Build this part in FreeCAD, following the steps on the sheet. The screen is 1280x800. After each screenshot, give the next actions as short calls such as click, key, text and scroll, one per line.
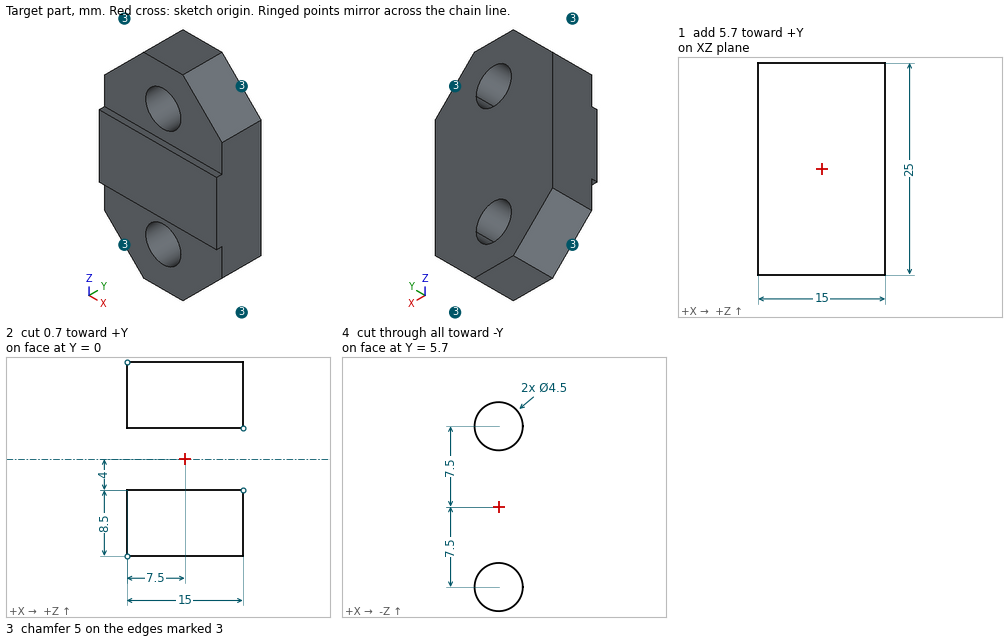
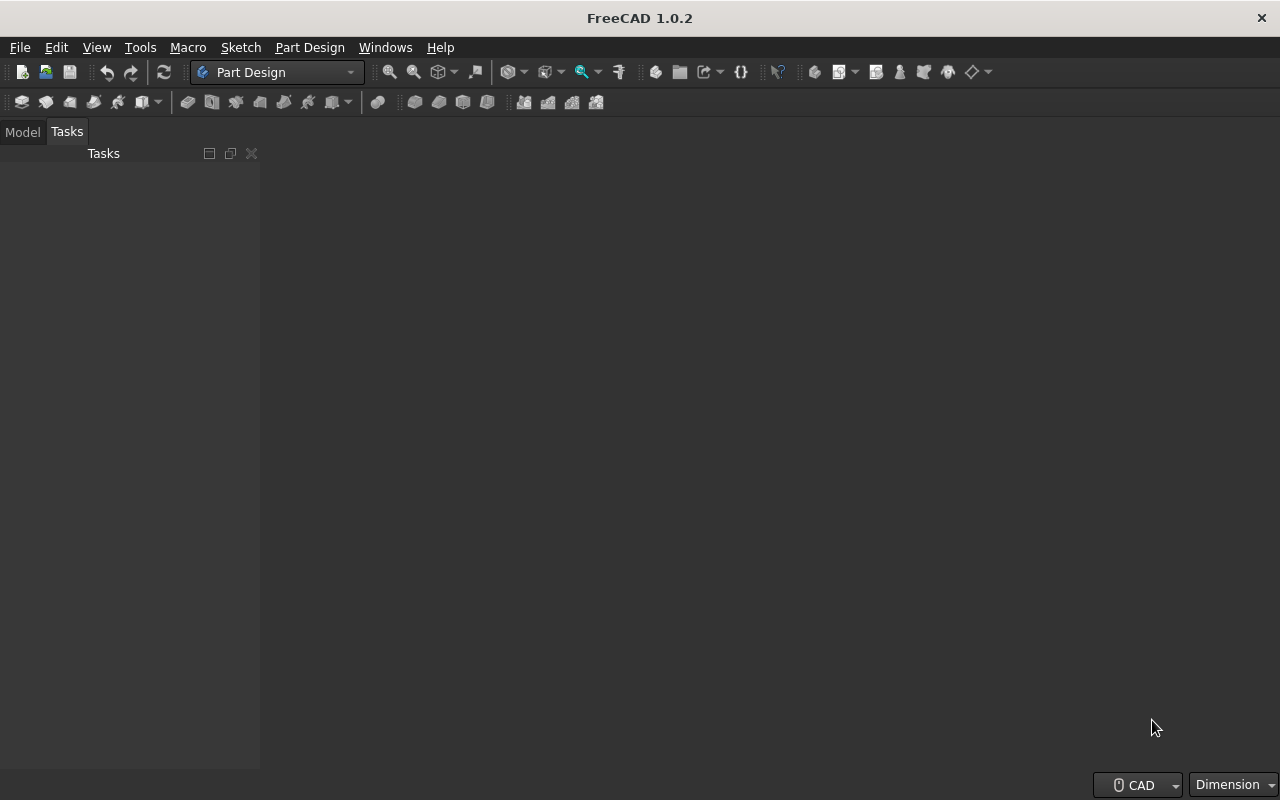
key(ctrl+n)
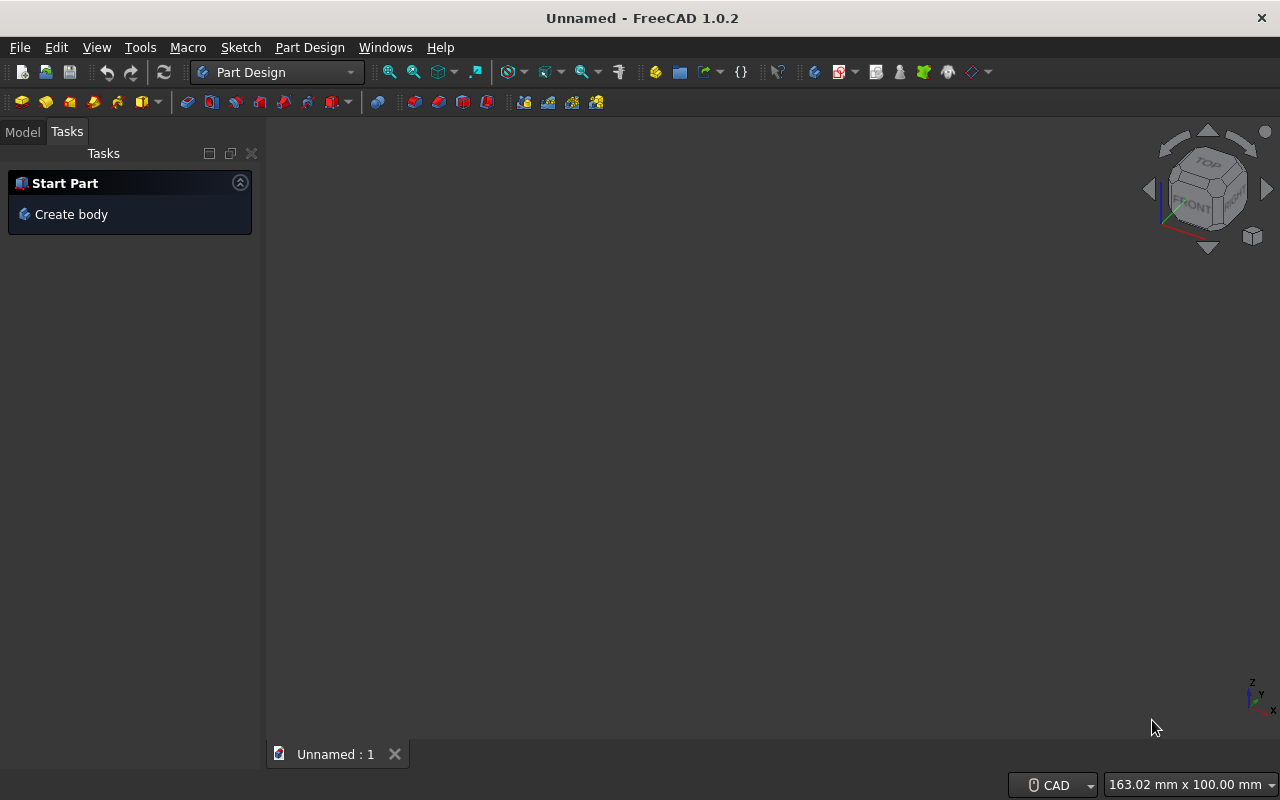
click(840, 72)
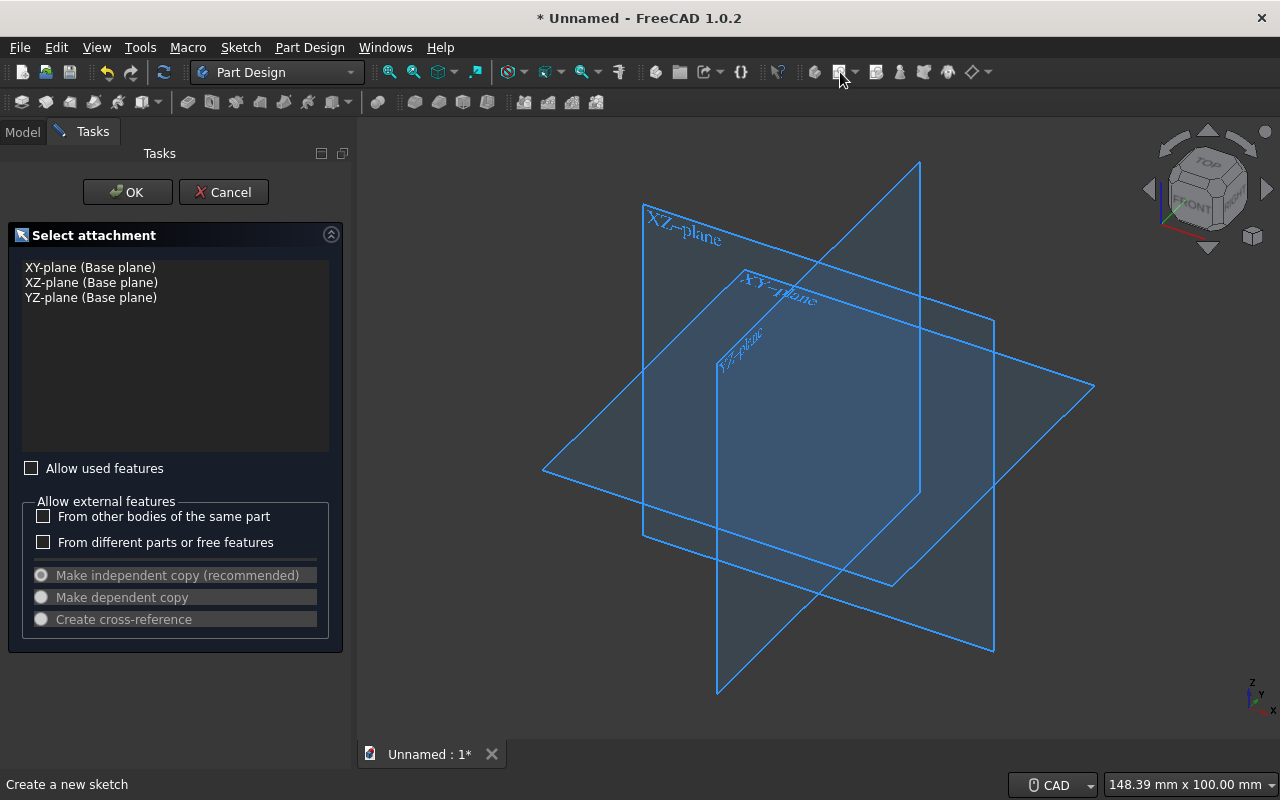
click(82, 282)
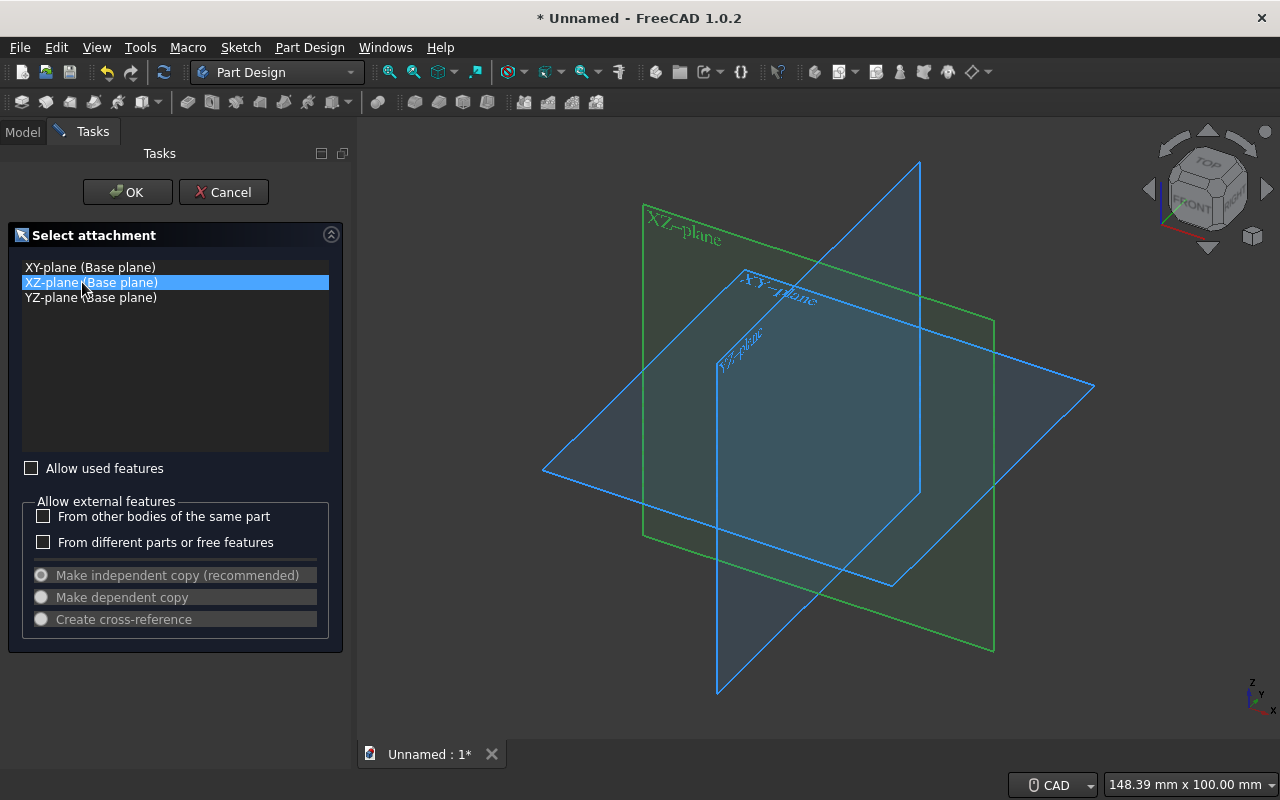
click(128, 192)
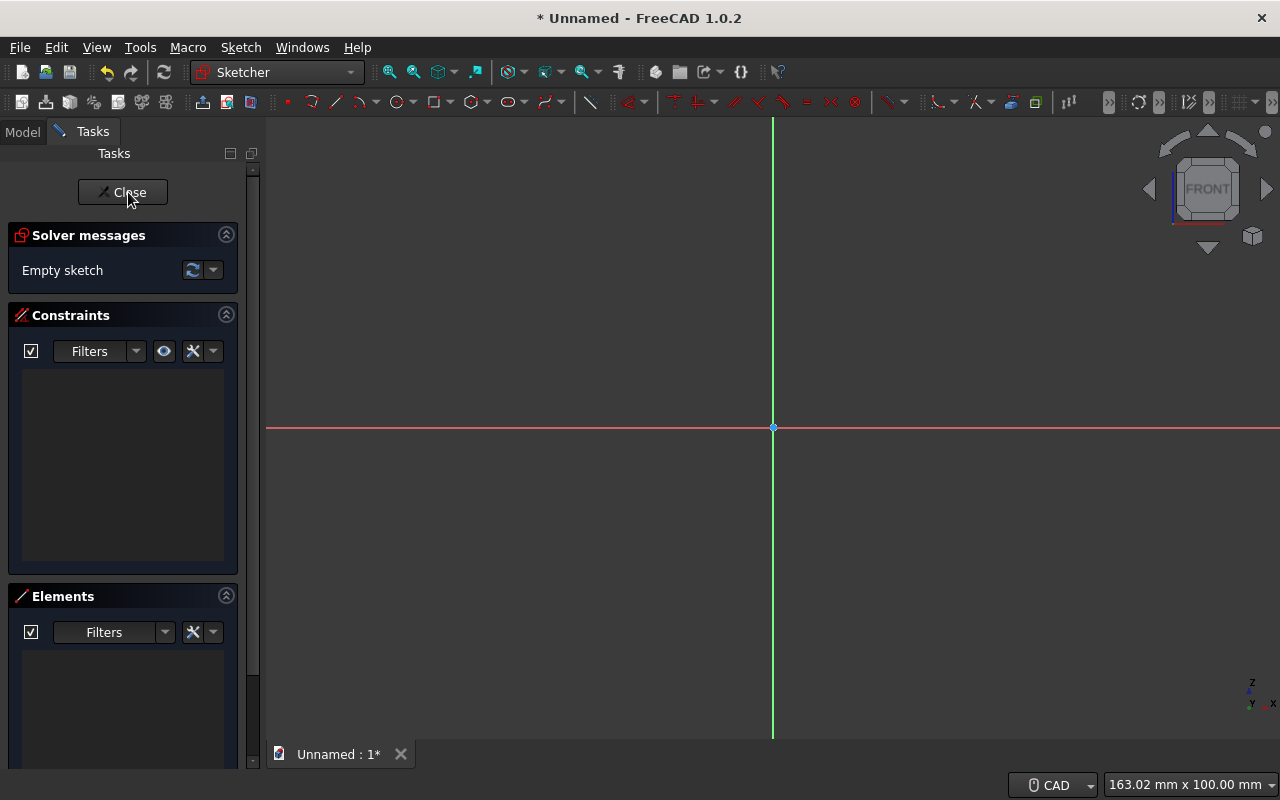
scroll(813, 428, up, 5)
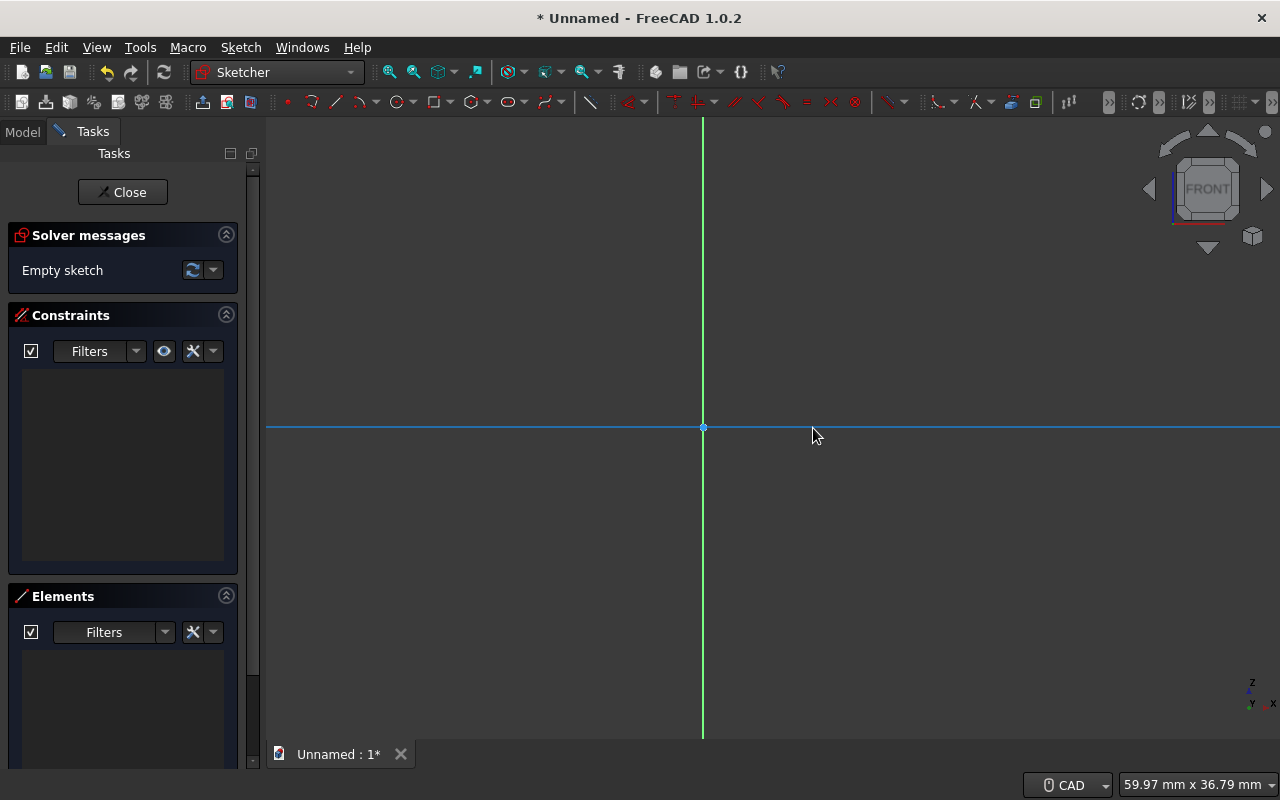
click(452, 102)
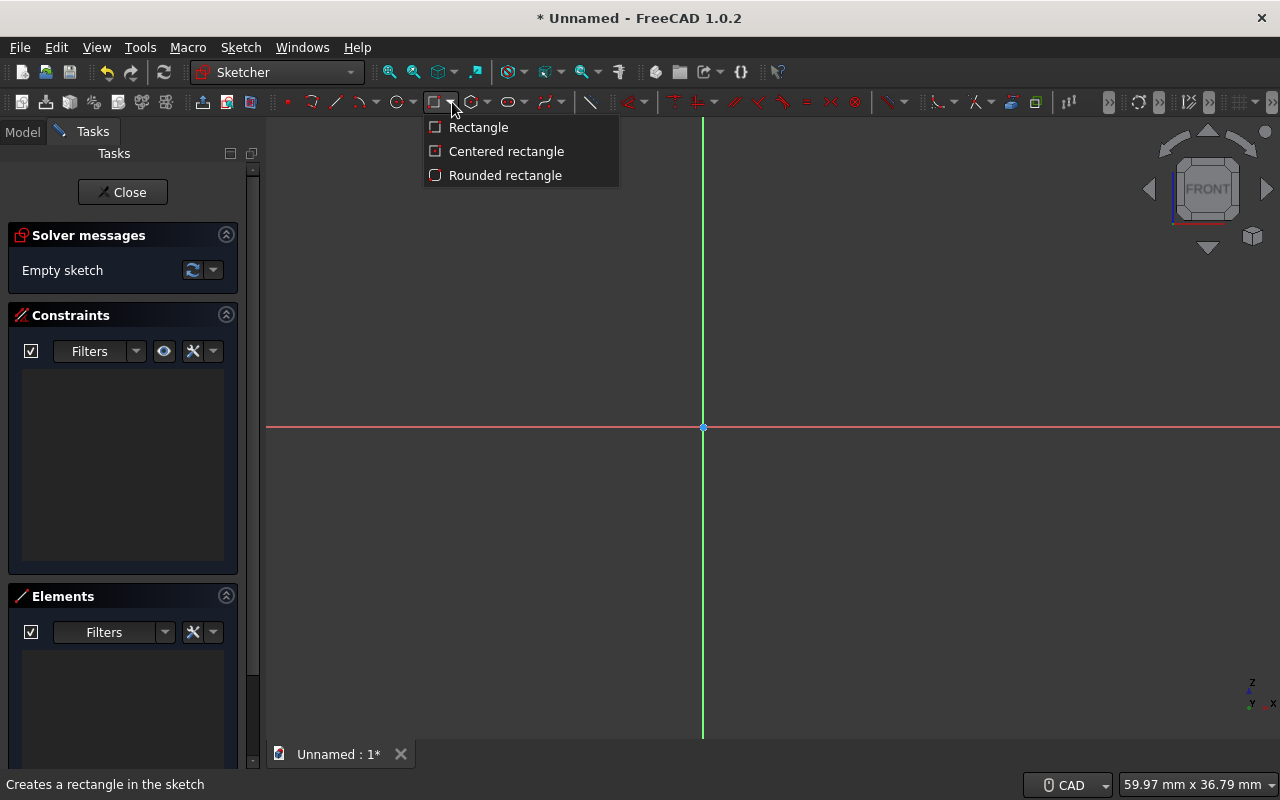
click(522, 151)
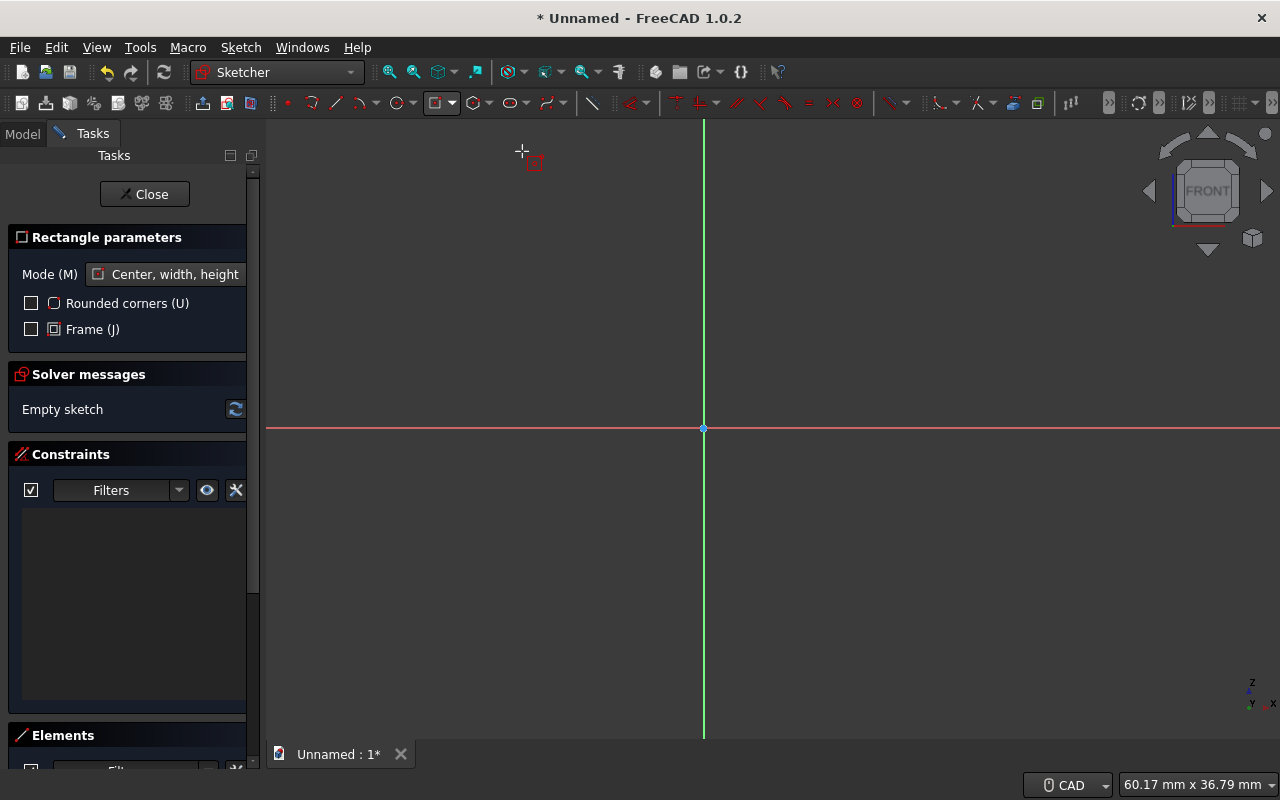
click(704, 428)
click(830, 217)
key(Escape)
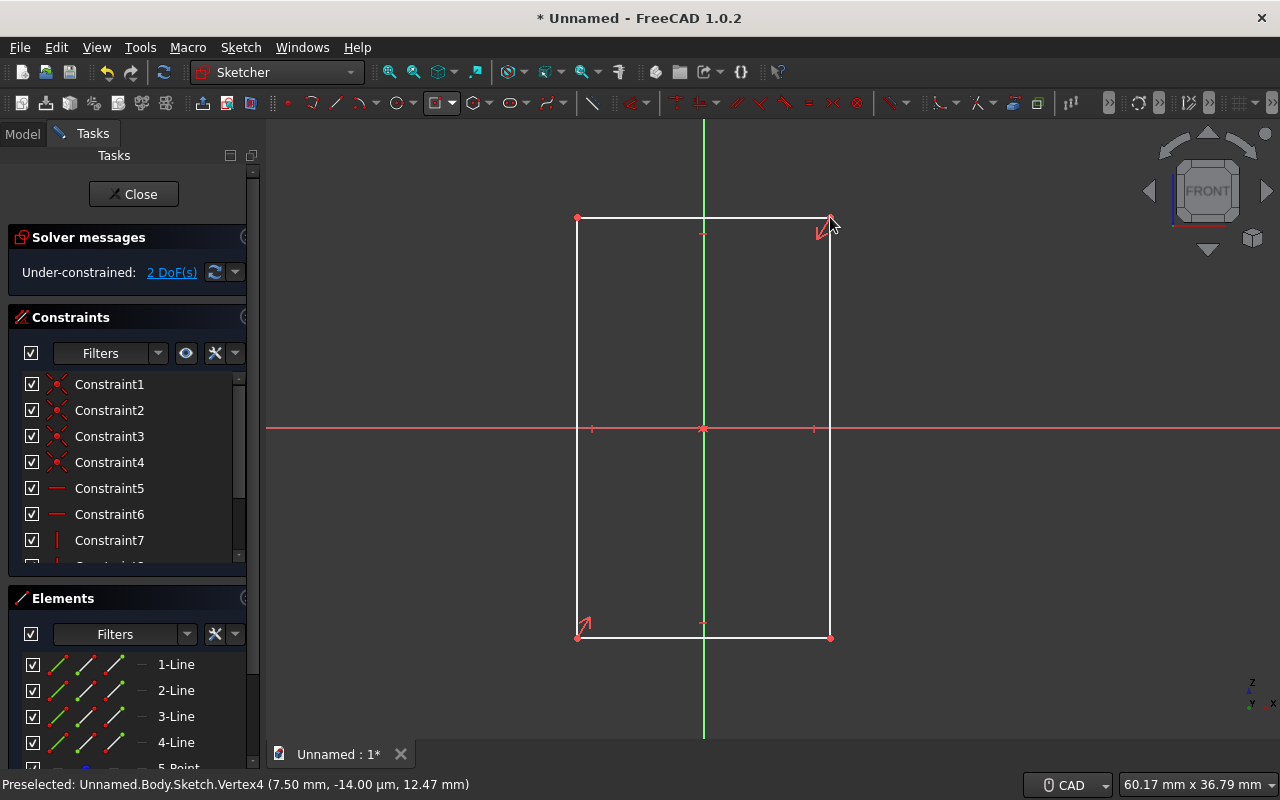
key(d)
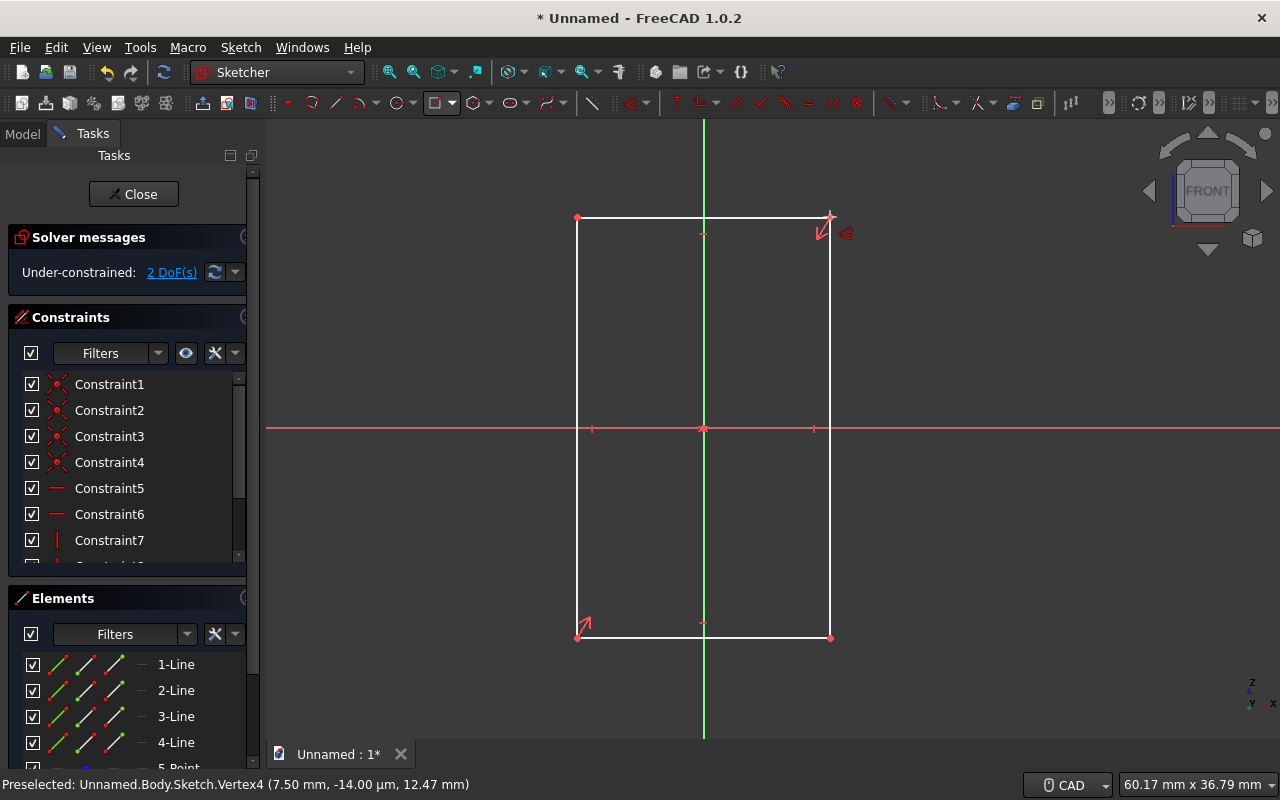
click(653, 638)
click(645, 672)